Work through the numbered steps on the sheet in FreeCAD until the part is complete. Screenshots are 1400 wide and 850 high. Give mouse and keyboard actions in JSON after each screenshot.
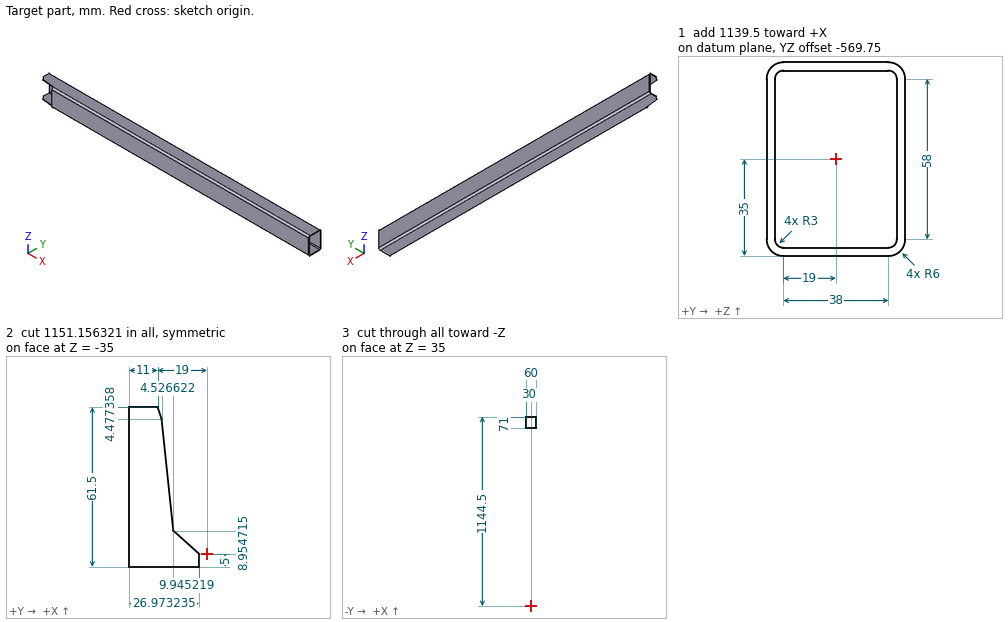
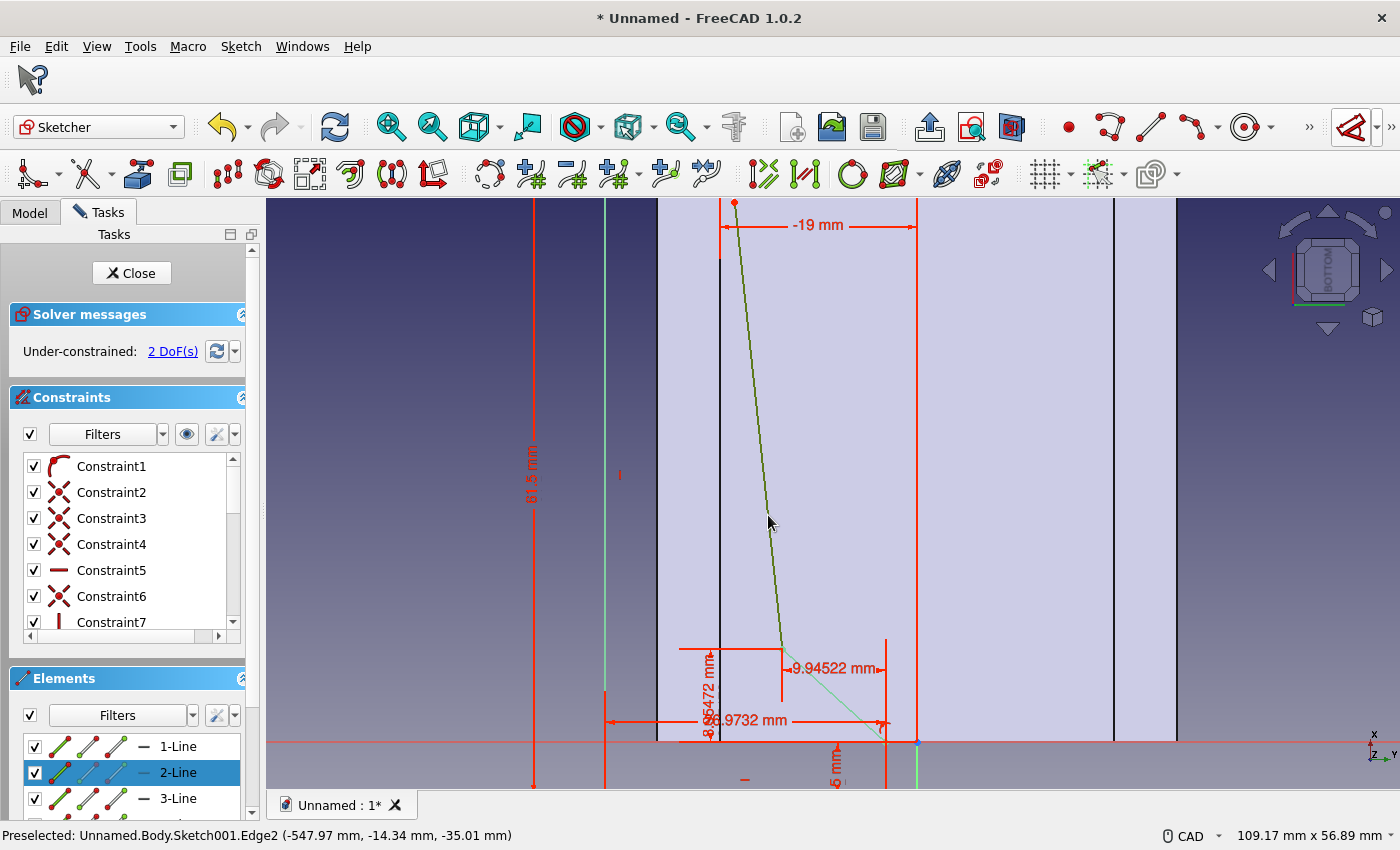
{"action": "key", "text": "l"}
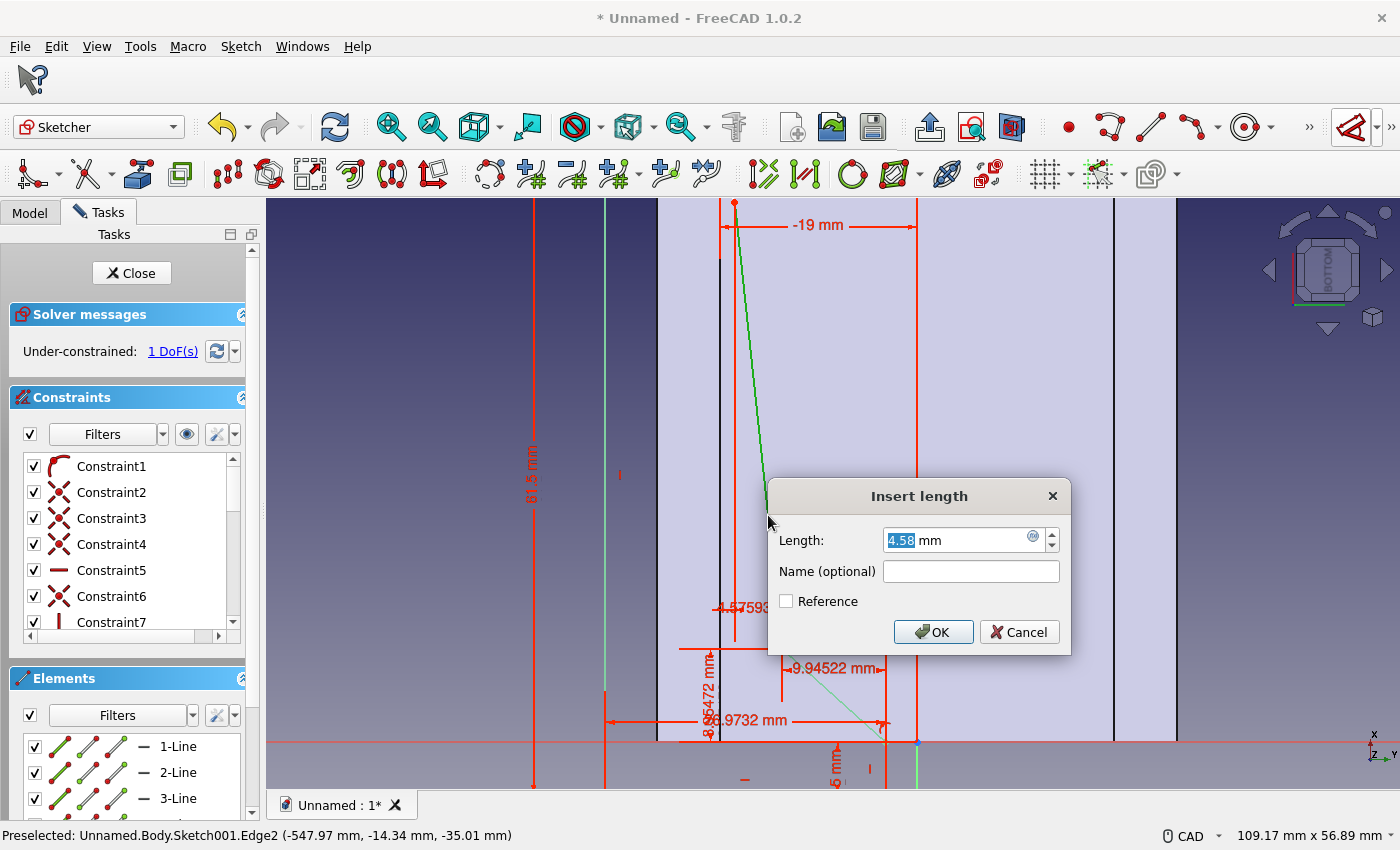
{"action": "type", "text": "4.526622"}
{"action": "key", "text": "Return"}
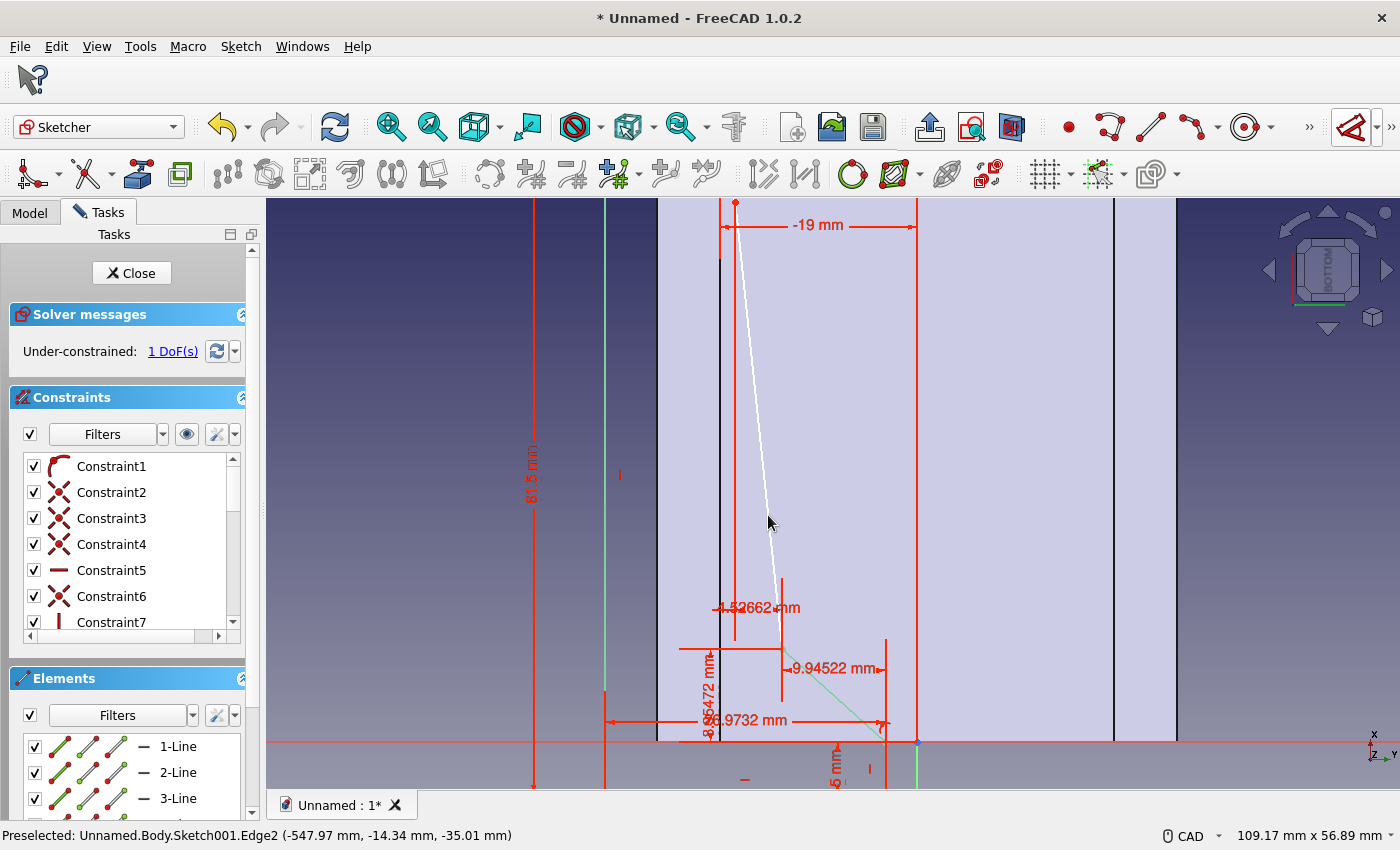
{"action": "scroll", "coordinate": [768, 516], "scroll_direction": "down", "scroll_amount": 3}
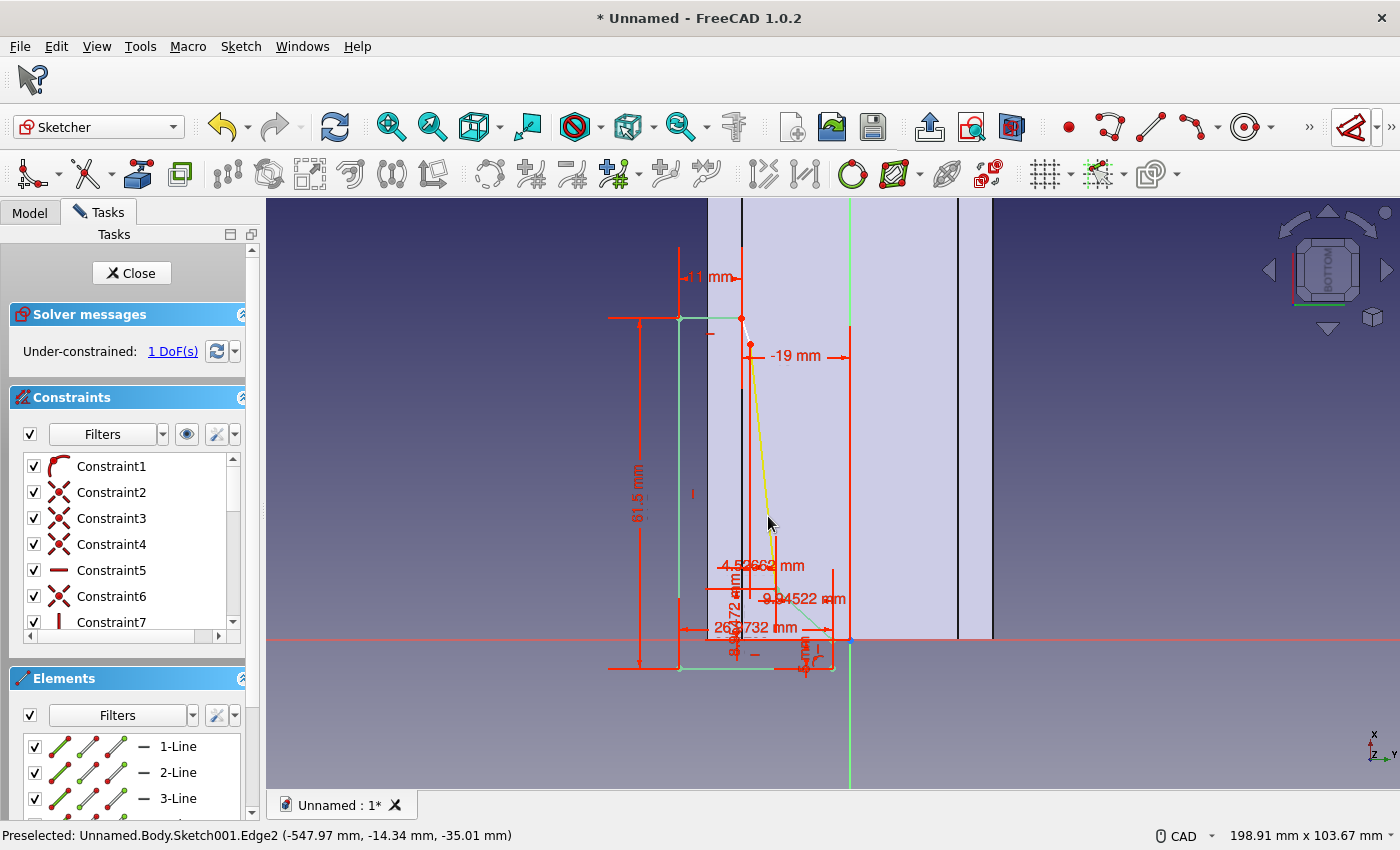
{"action": "scroll", "coordinate": [748, 337], "scroll_direction": "up", "scroll_amount": 3}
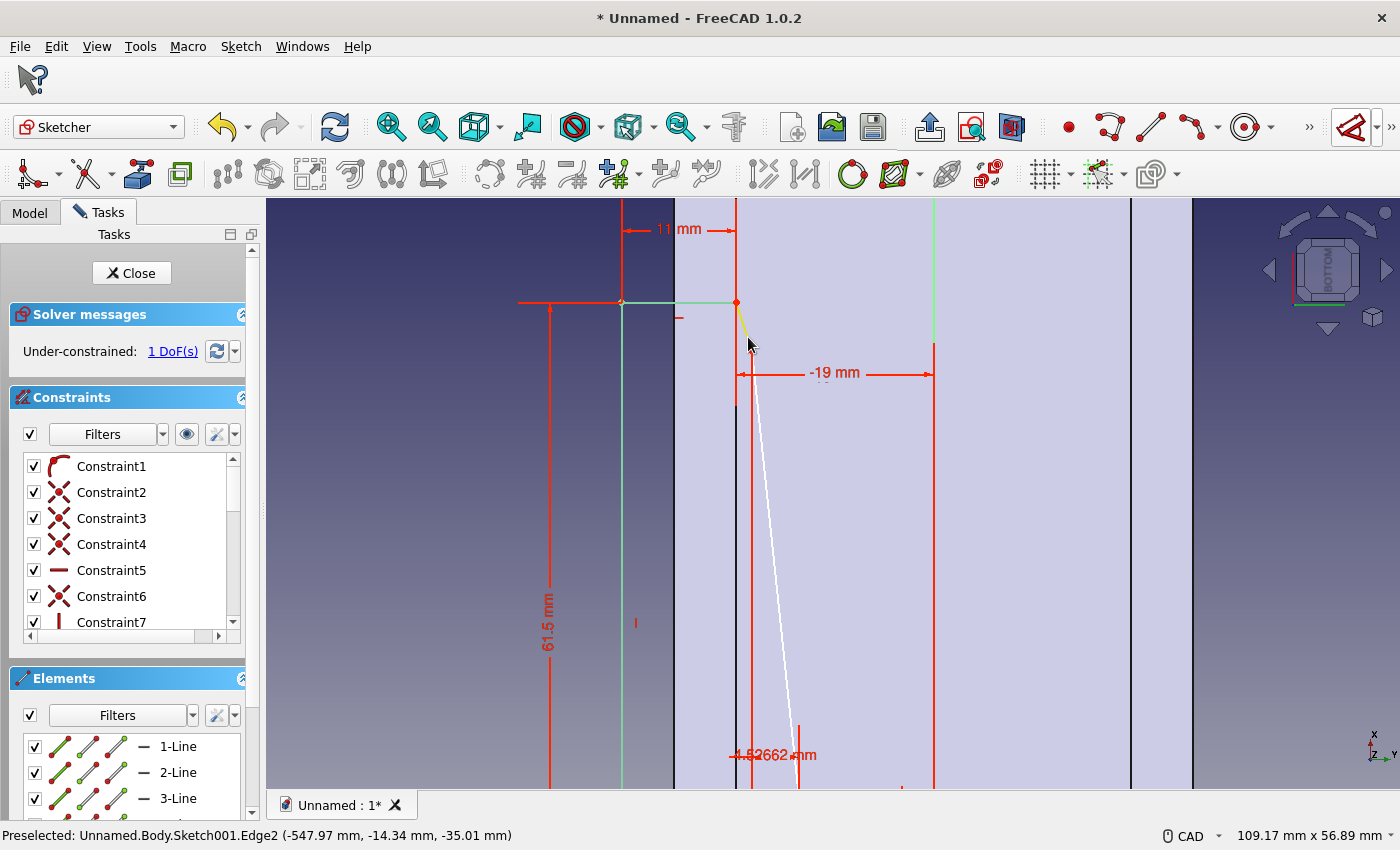
{"action": "left_click", "coordinate": [747, 336]}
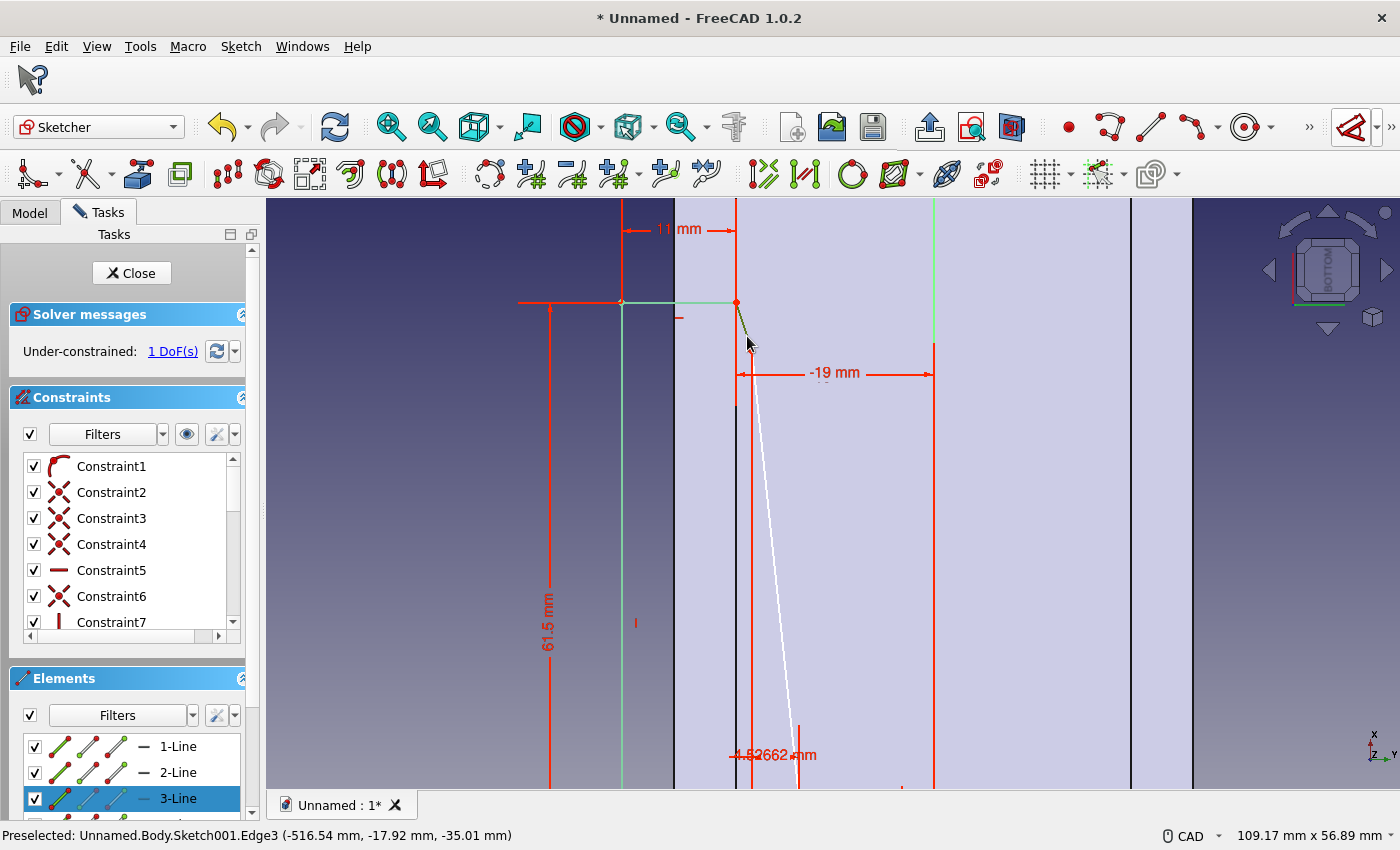
{"action": "key", "text": "i"}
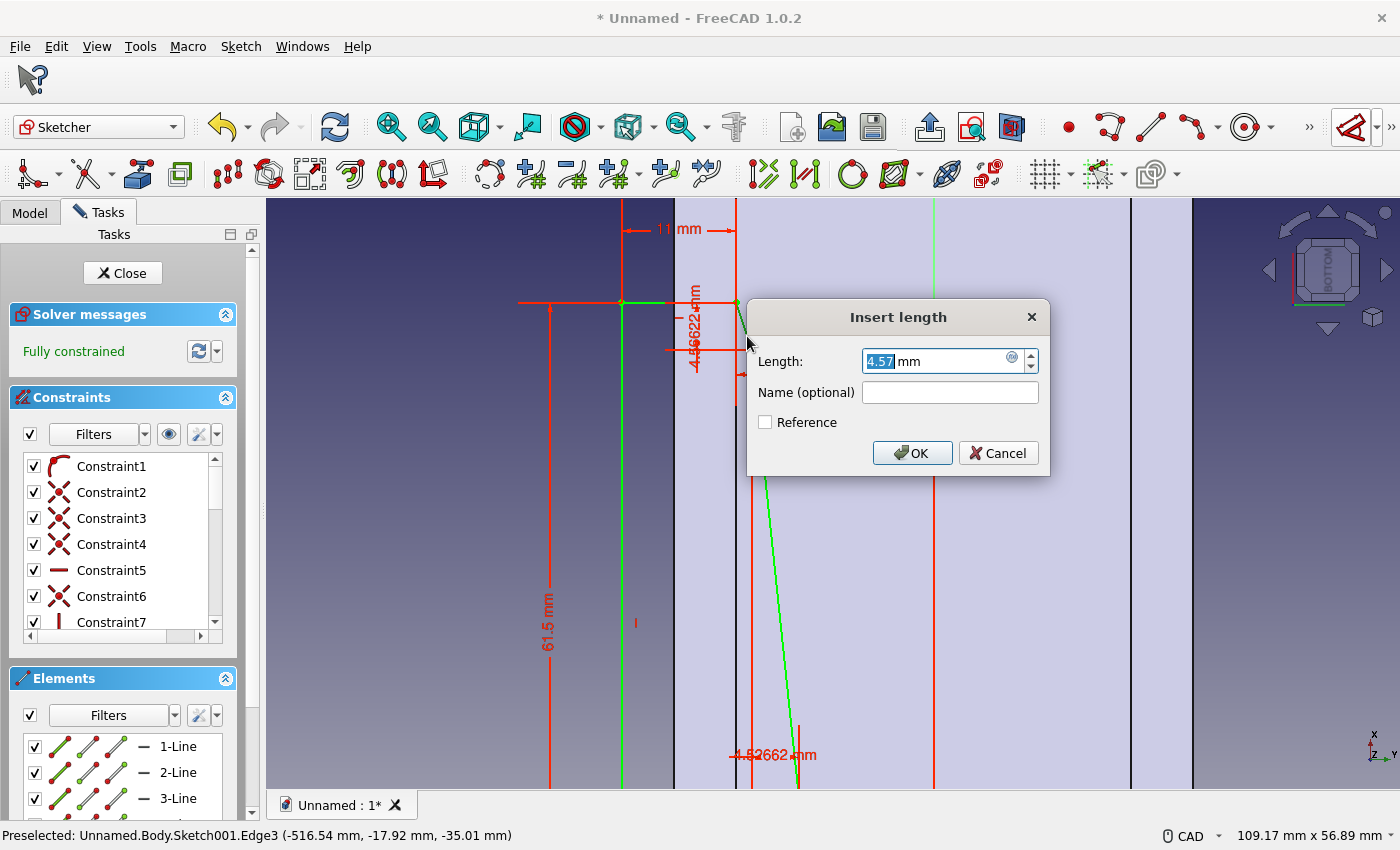
{"action": "type", "text": "4.477358"}
{"action": "key", "text": "Return"}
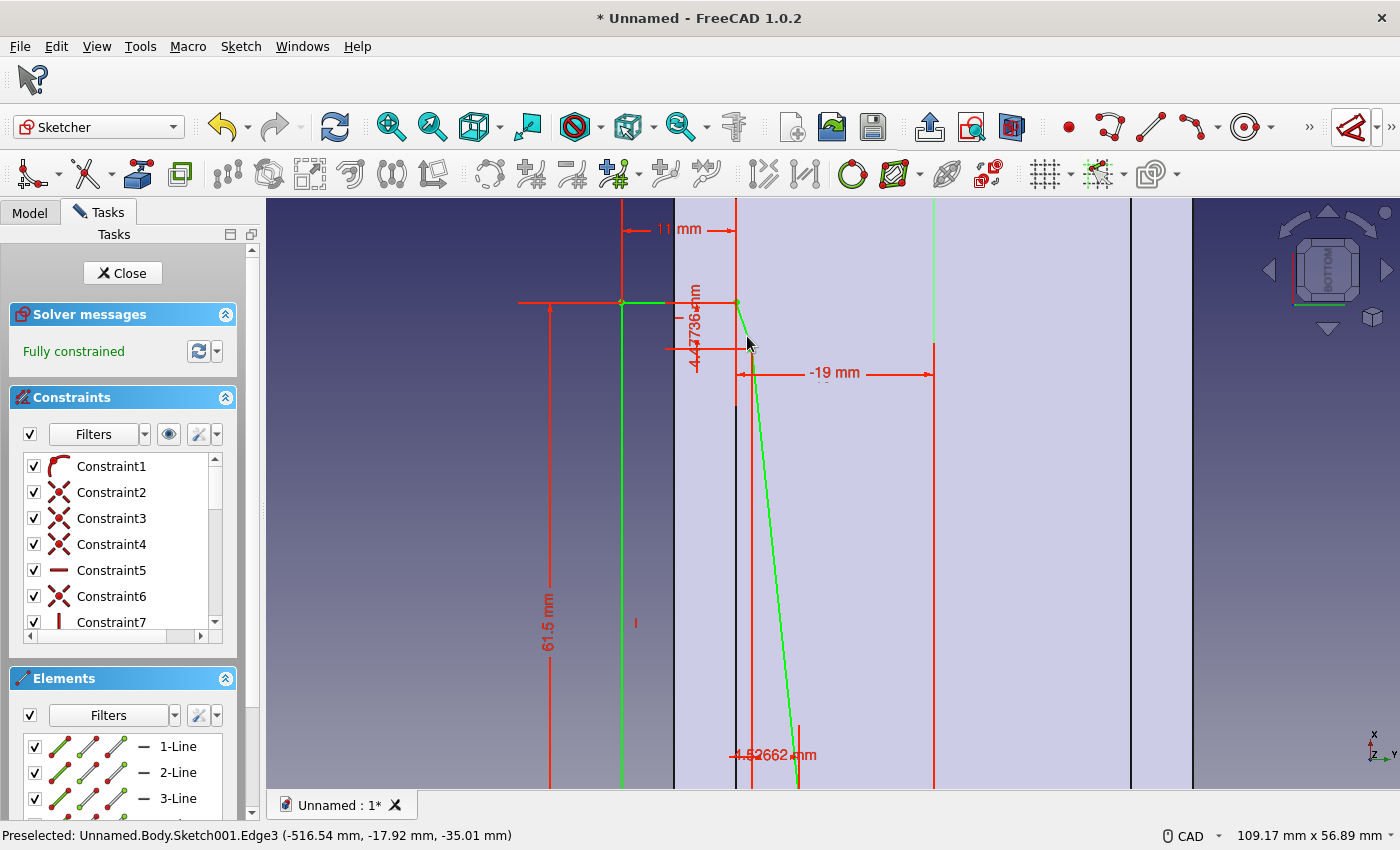
{"action": "left_click", "coordinate": [123, 273]}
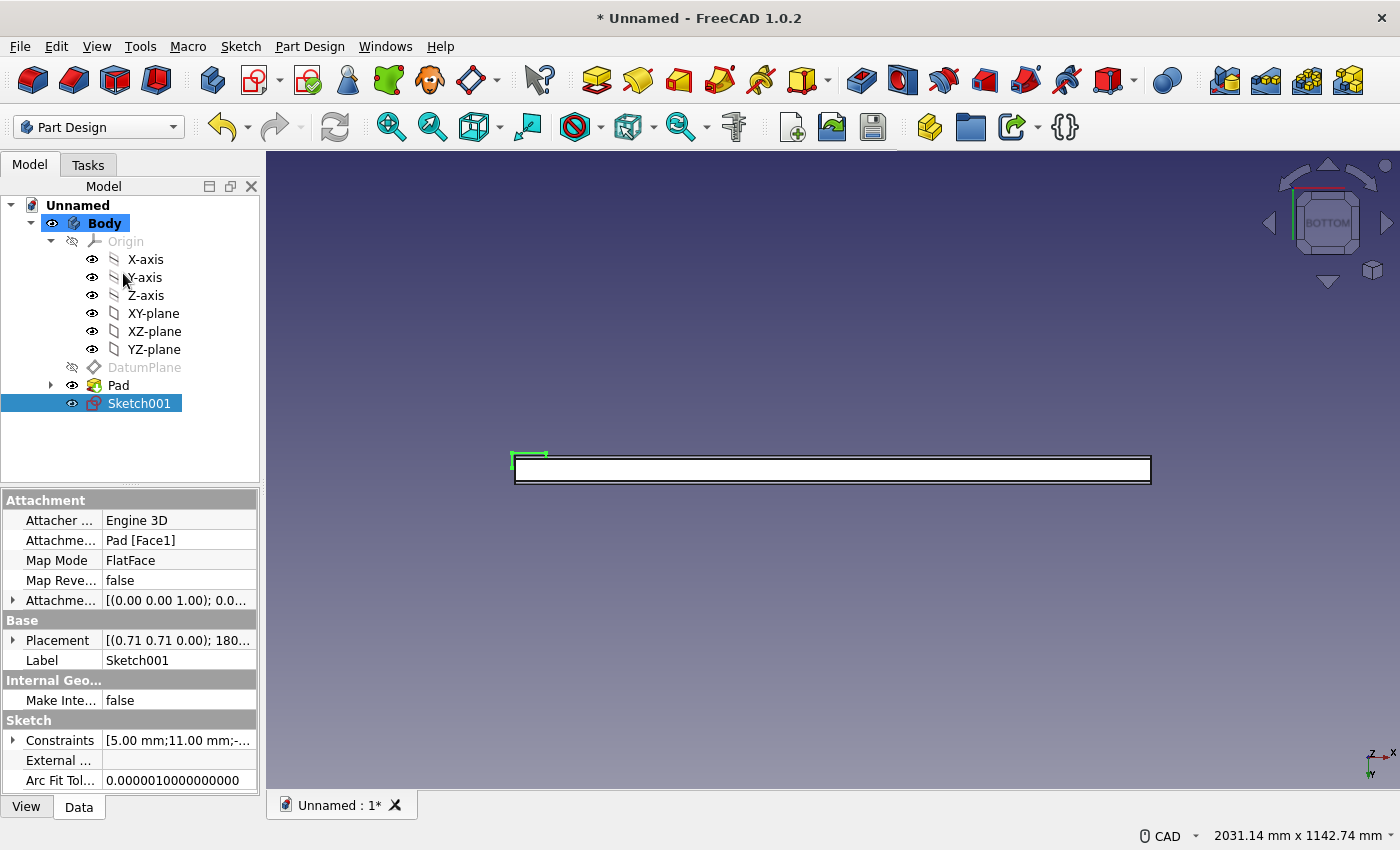
{"action": "left_click", "coordinate": [862, 80]}